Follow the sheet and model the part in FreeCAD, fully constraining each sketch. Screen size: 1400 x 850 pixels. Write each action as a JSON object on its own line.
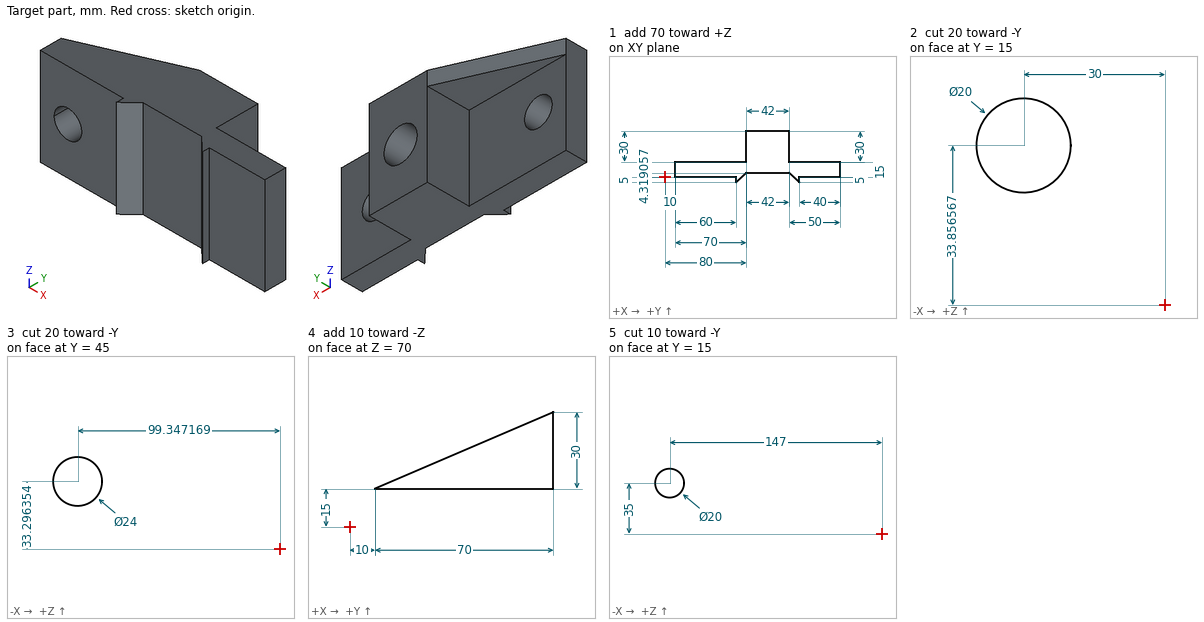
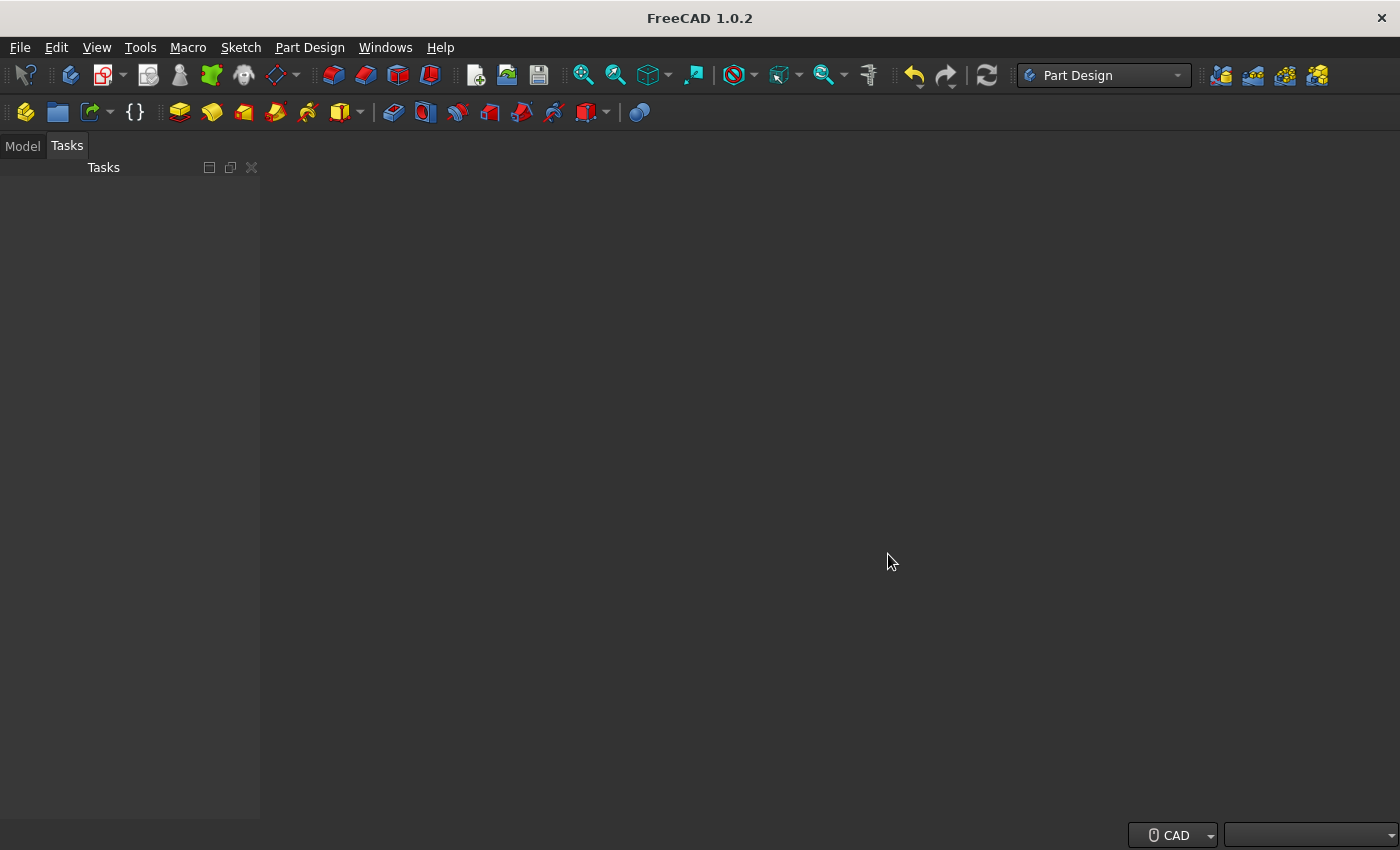
{"action": "left_click", "coordinate": [476, 76]}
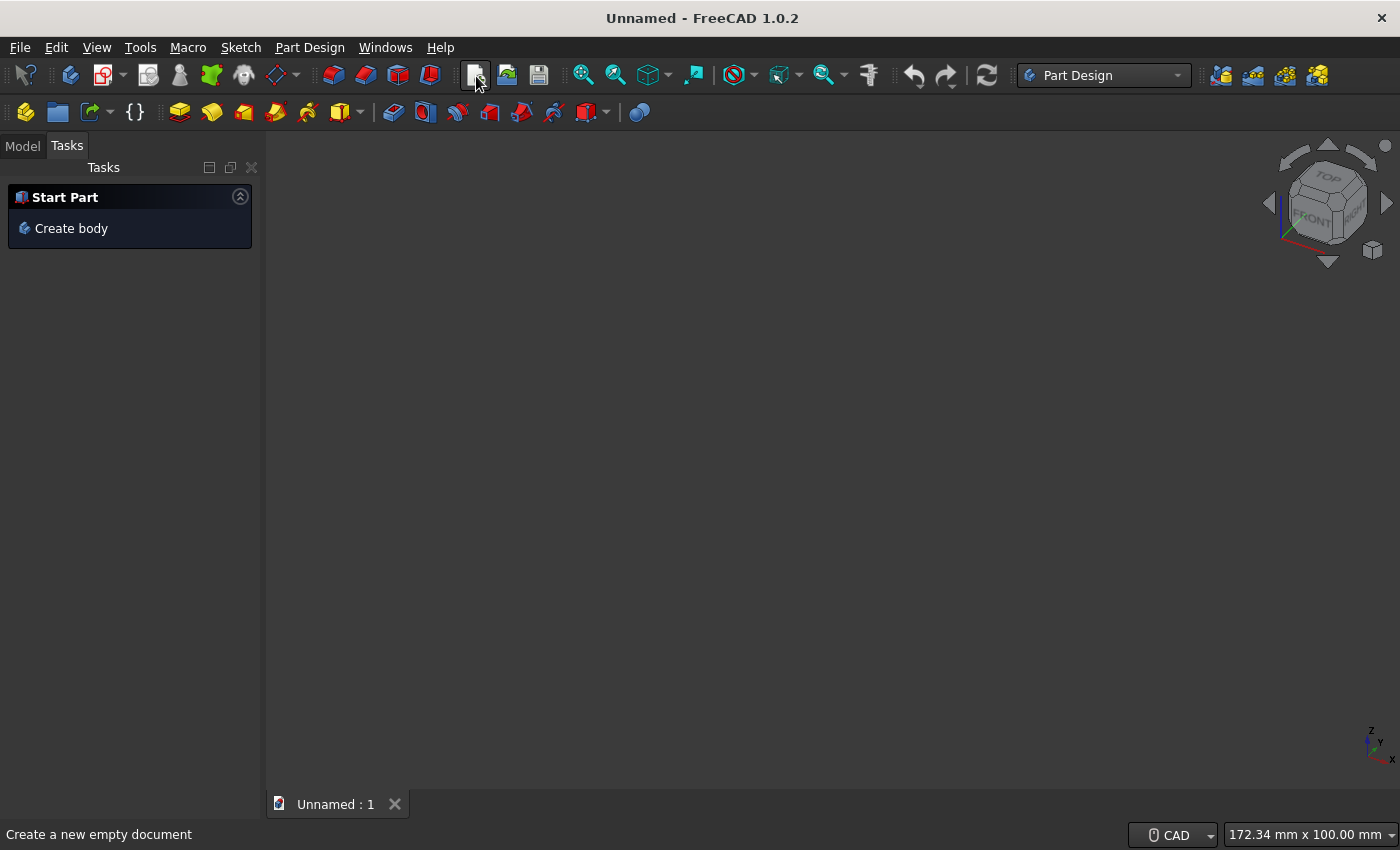
{"action": "left_click", "coordinate": [104, 76]}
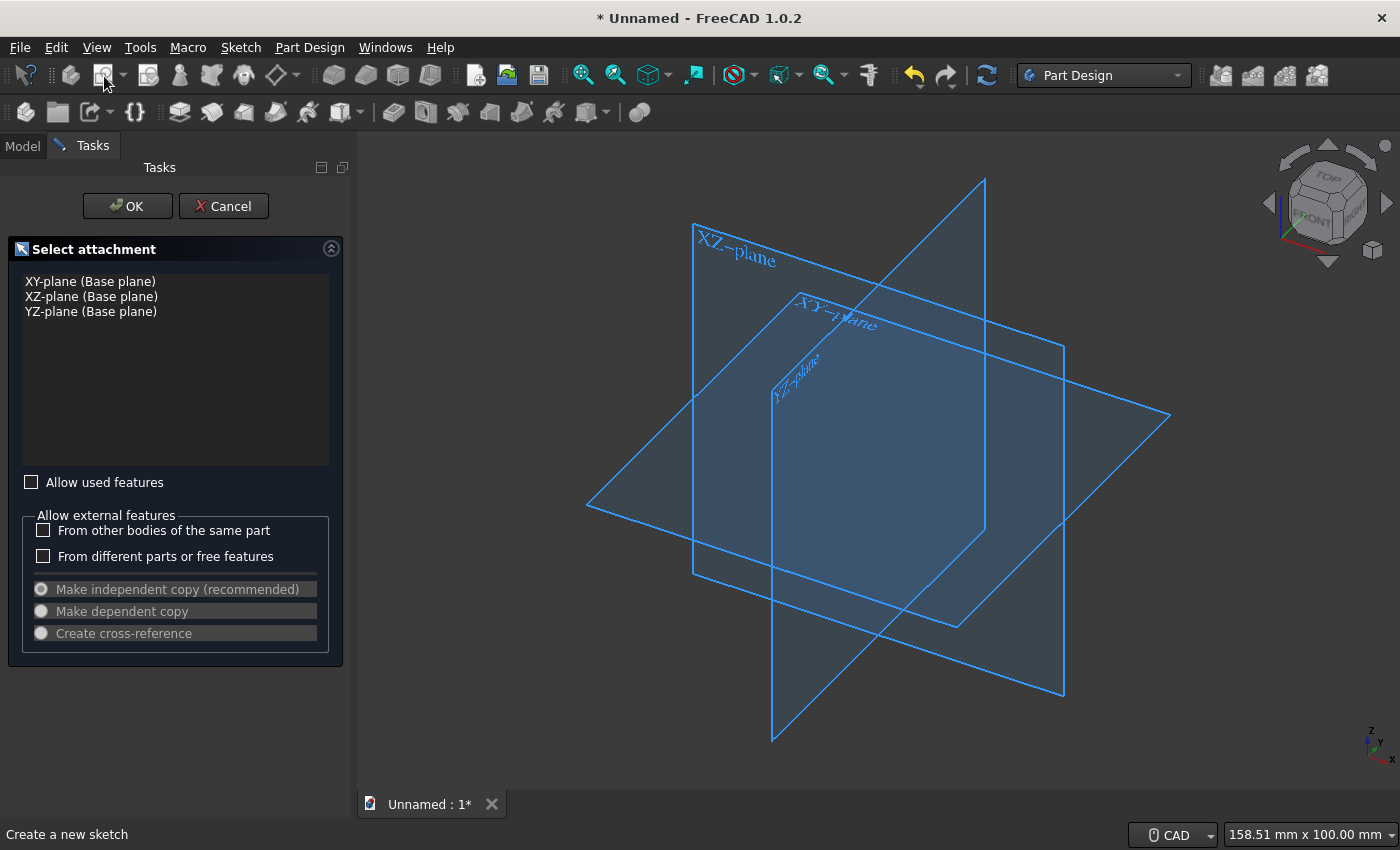
{"action": "left_click", "coordinate": [82, 282]}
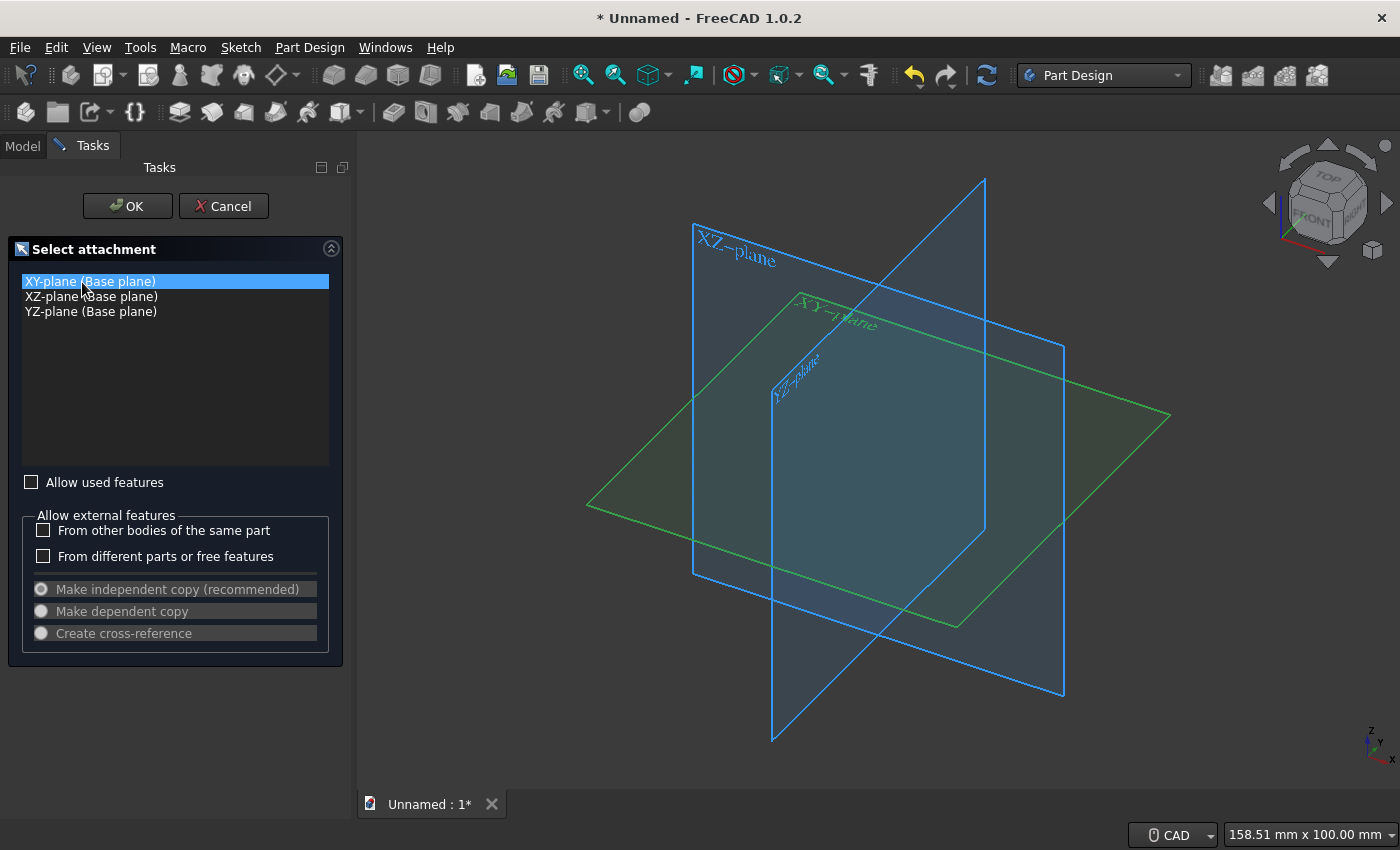
{"action": "left_click", "coordinate": [128, 206]}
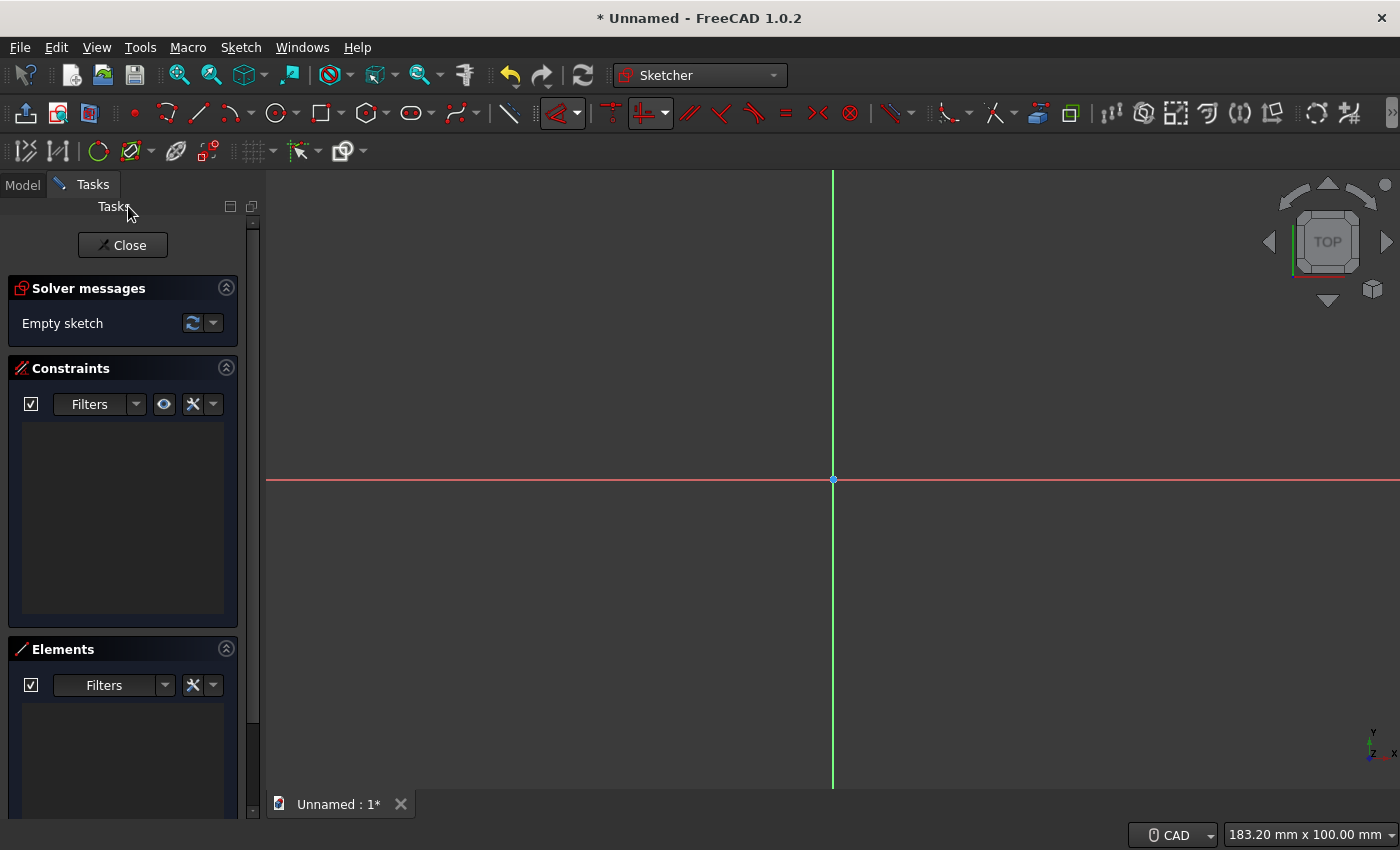
{"action": "scroll", "coordinate": [294, 630], "scroll_direction": "down", "scroll_amount": 3}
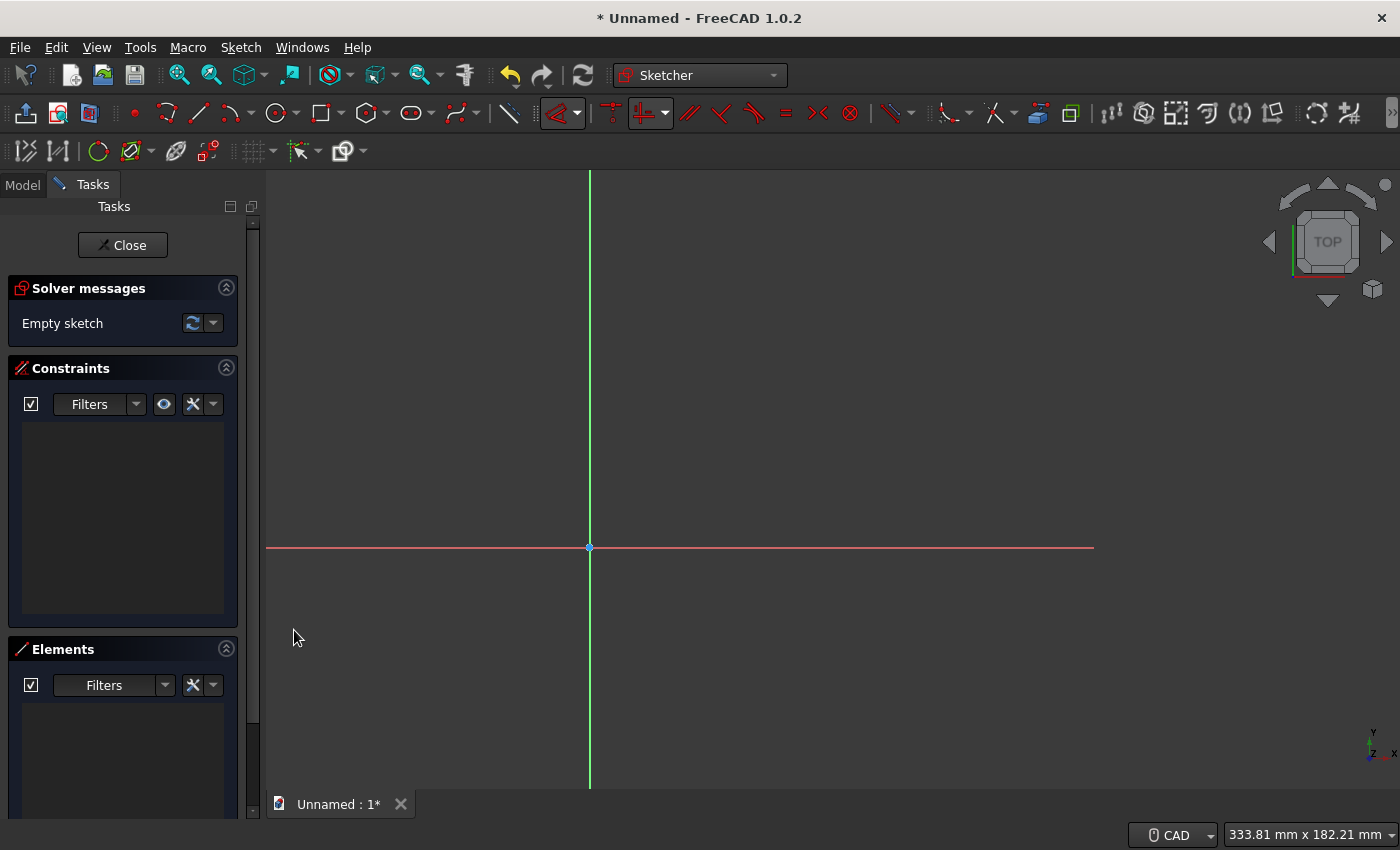
{"action": "left_click", "coordinate": [168, 114]}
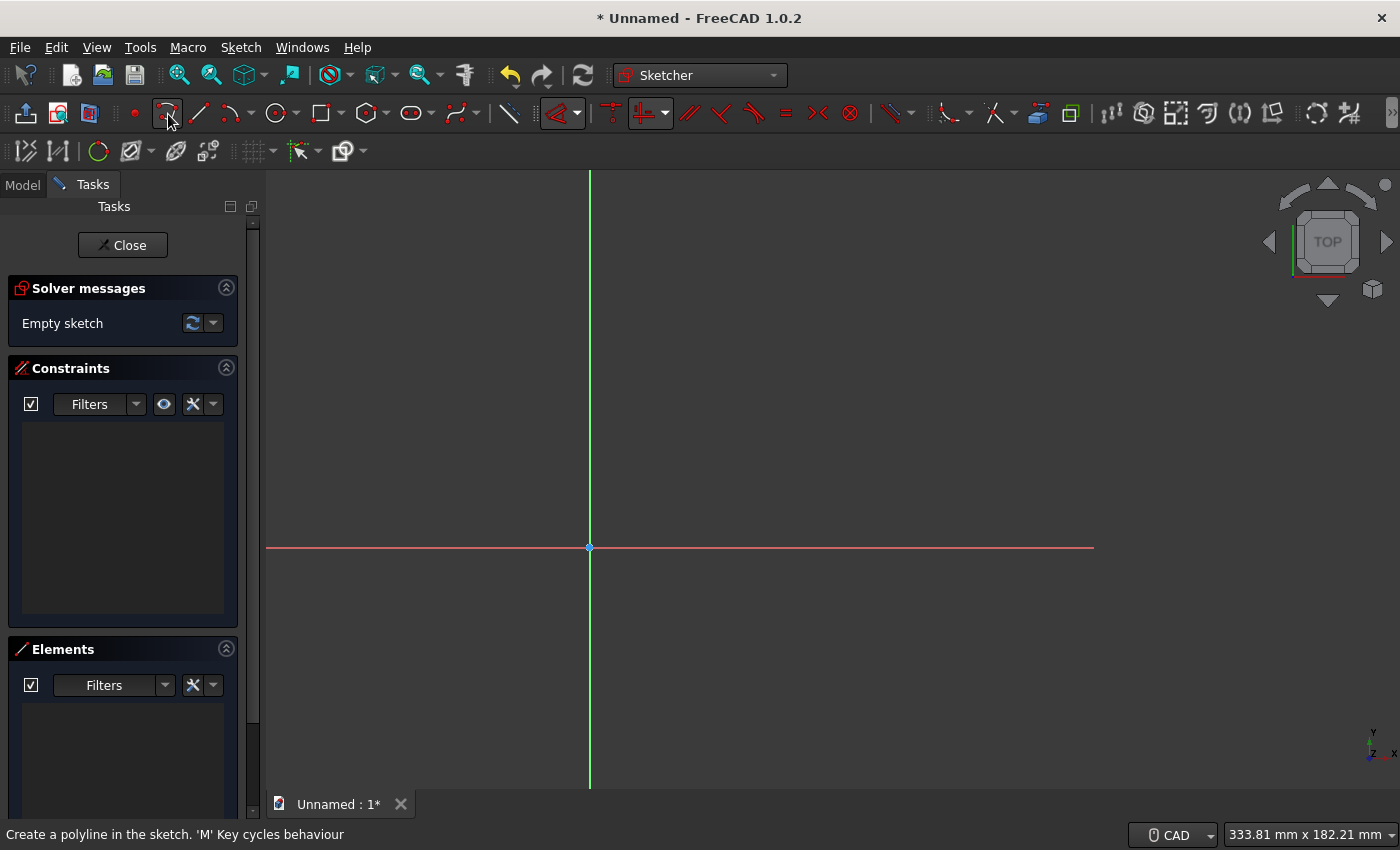
{"action": "left_click", "coordinate": [624, 548]}
{"action": "left_click", "coordinate": [828, 539]}
{"action": "left_click", "coordinate": [828, 565]}
{"action": "left_click", "coordinate": [862, 533]}
{"action": "left_click", "coordinate": [1004, 533]}
{"action": "left_click", "coordinate": [1038, 565]}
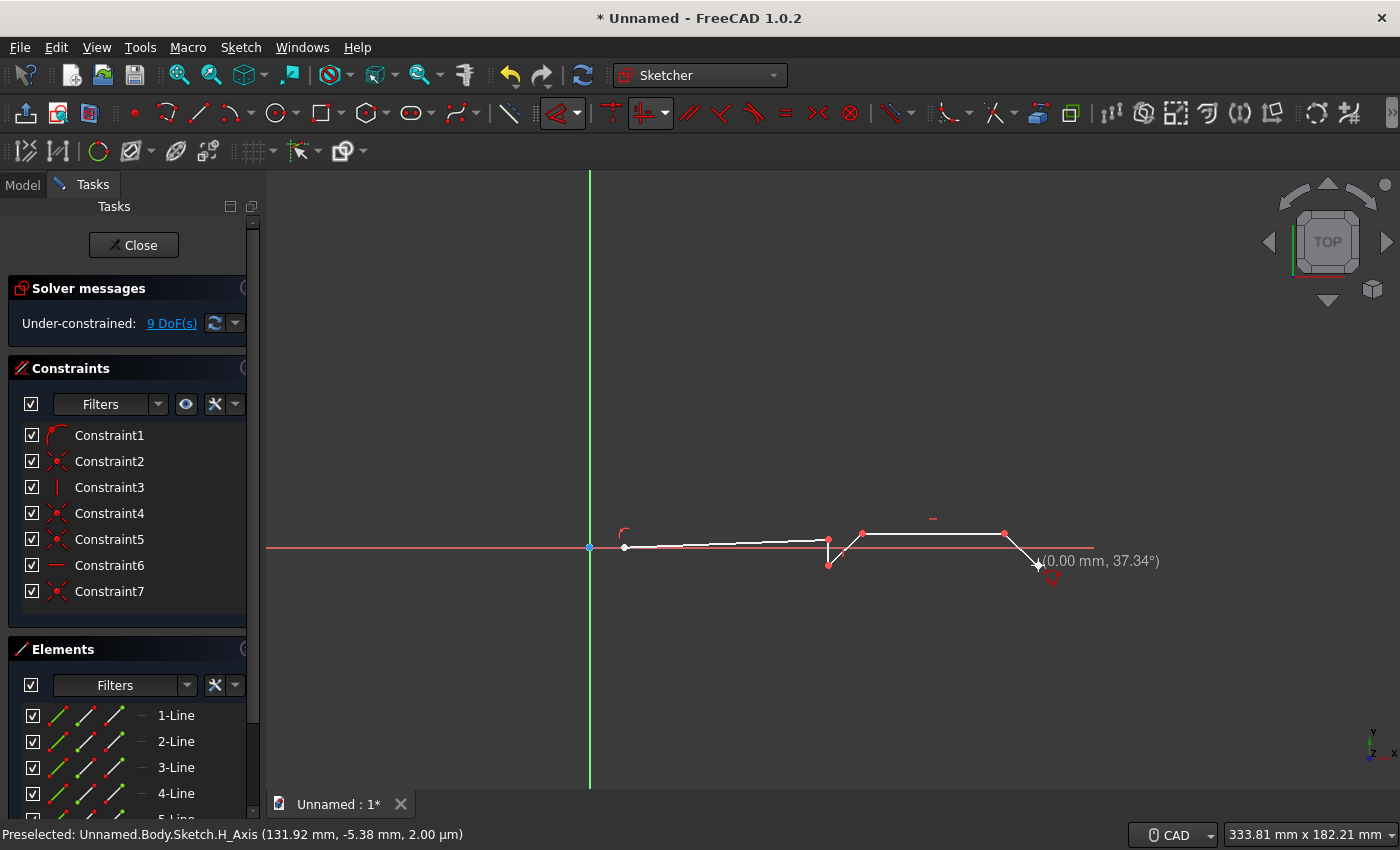
{"action": "scroll", "coordinate": [1038, 548], "scroll_direction": "up", "scroll_amount": 2}